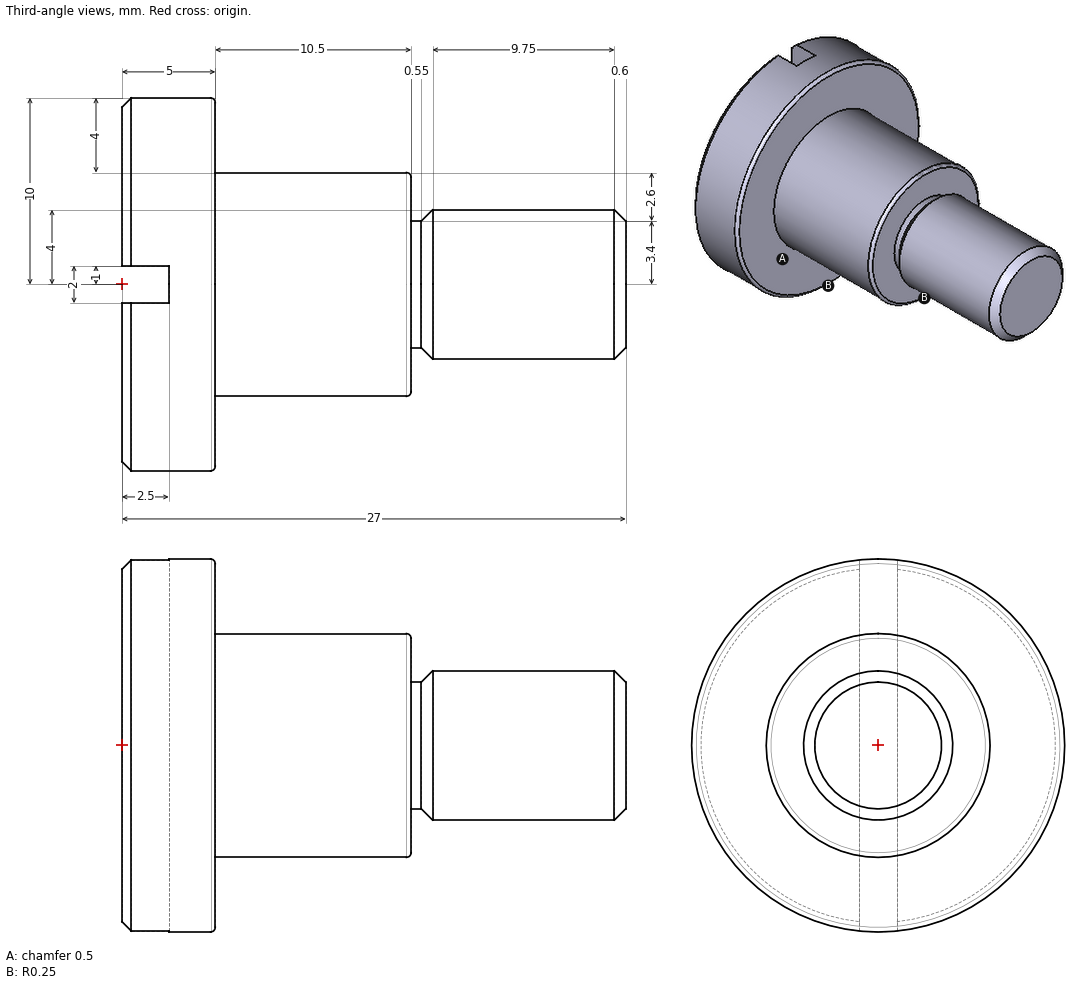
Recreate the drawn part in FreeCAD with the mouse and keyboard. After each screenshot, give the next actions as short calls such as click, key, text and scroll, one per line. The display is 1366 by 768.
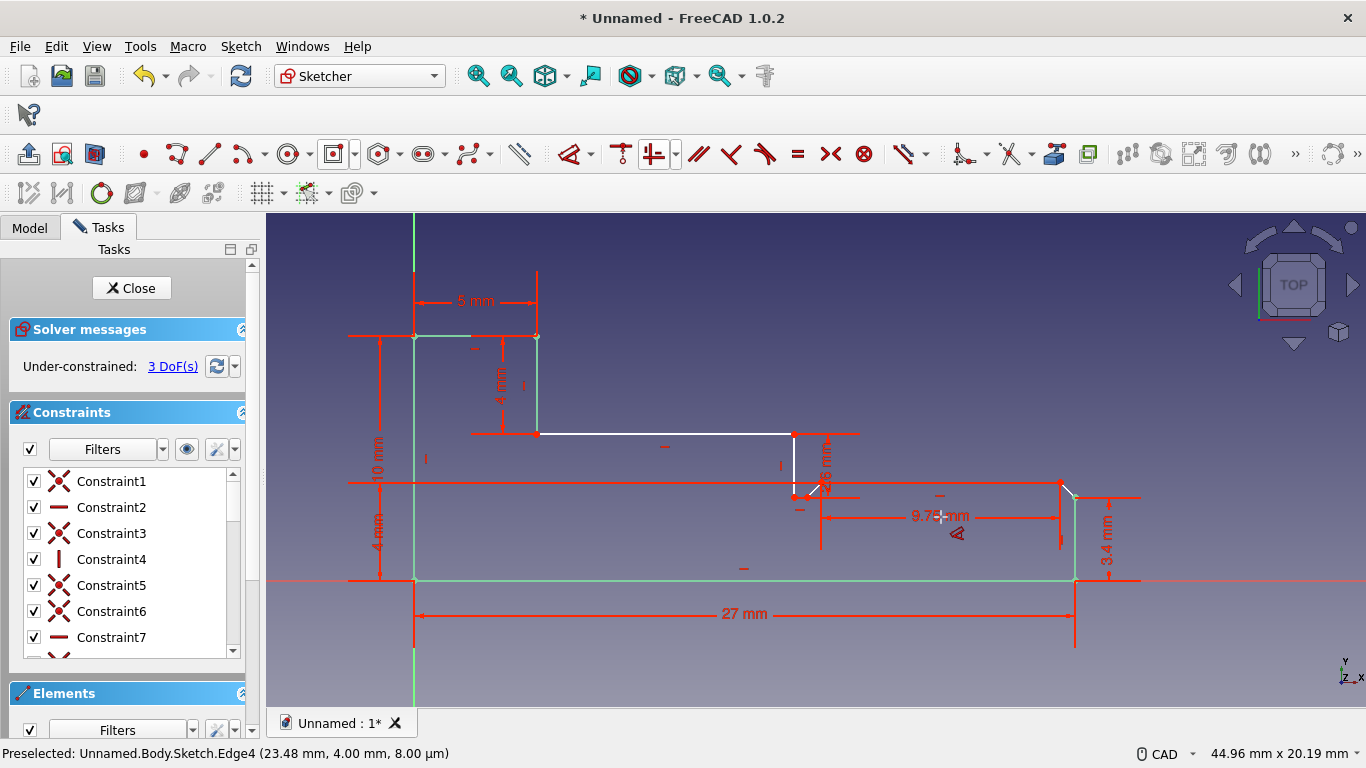
scroll(801, 498, up, 6)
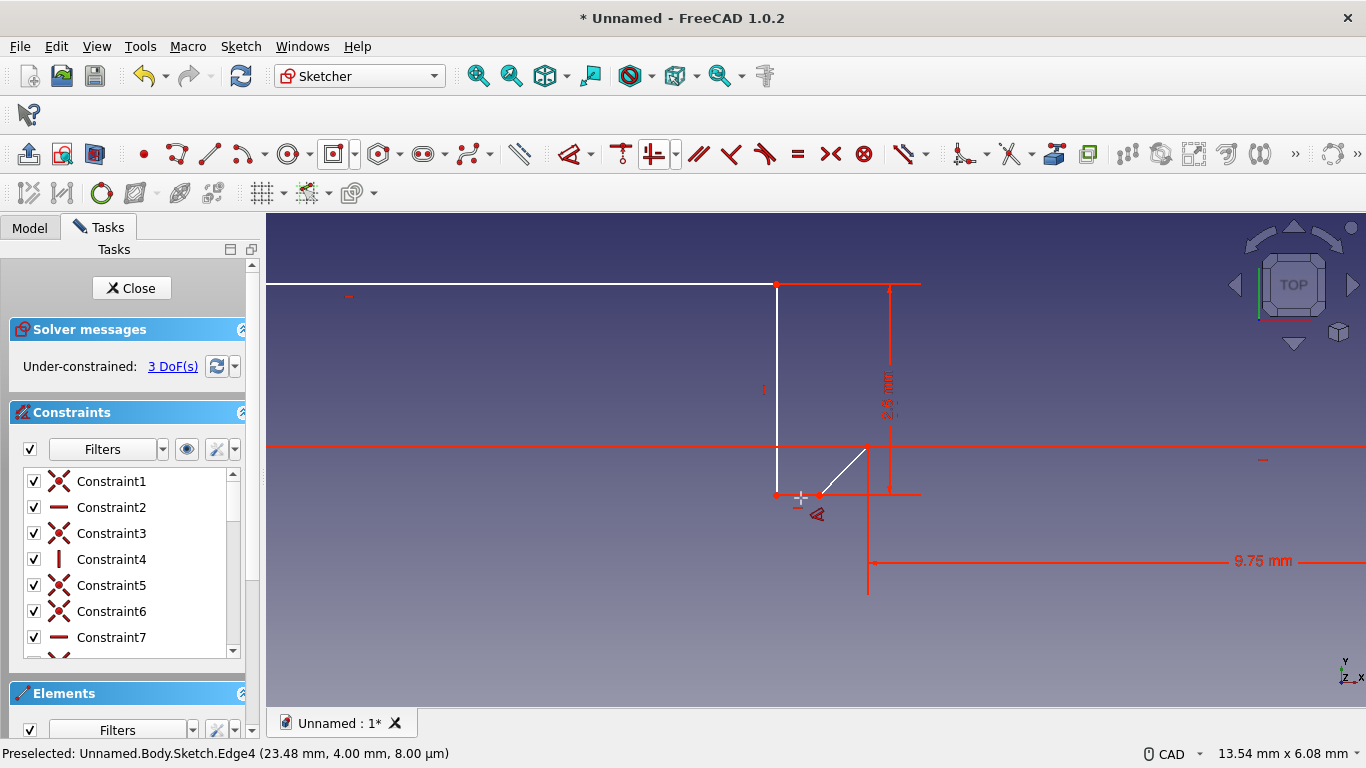
click(798, 495)
click(798, 529)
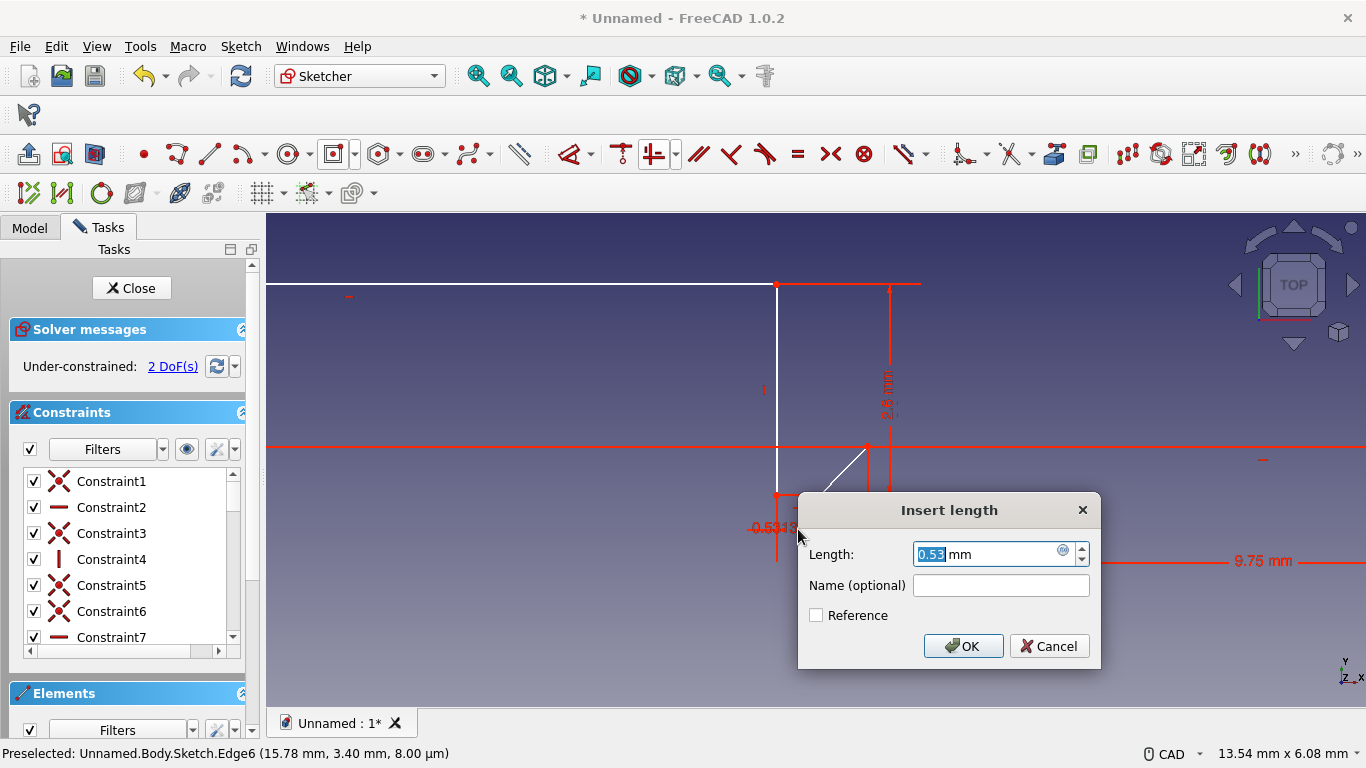
text(0.55)
key(Return)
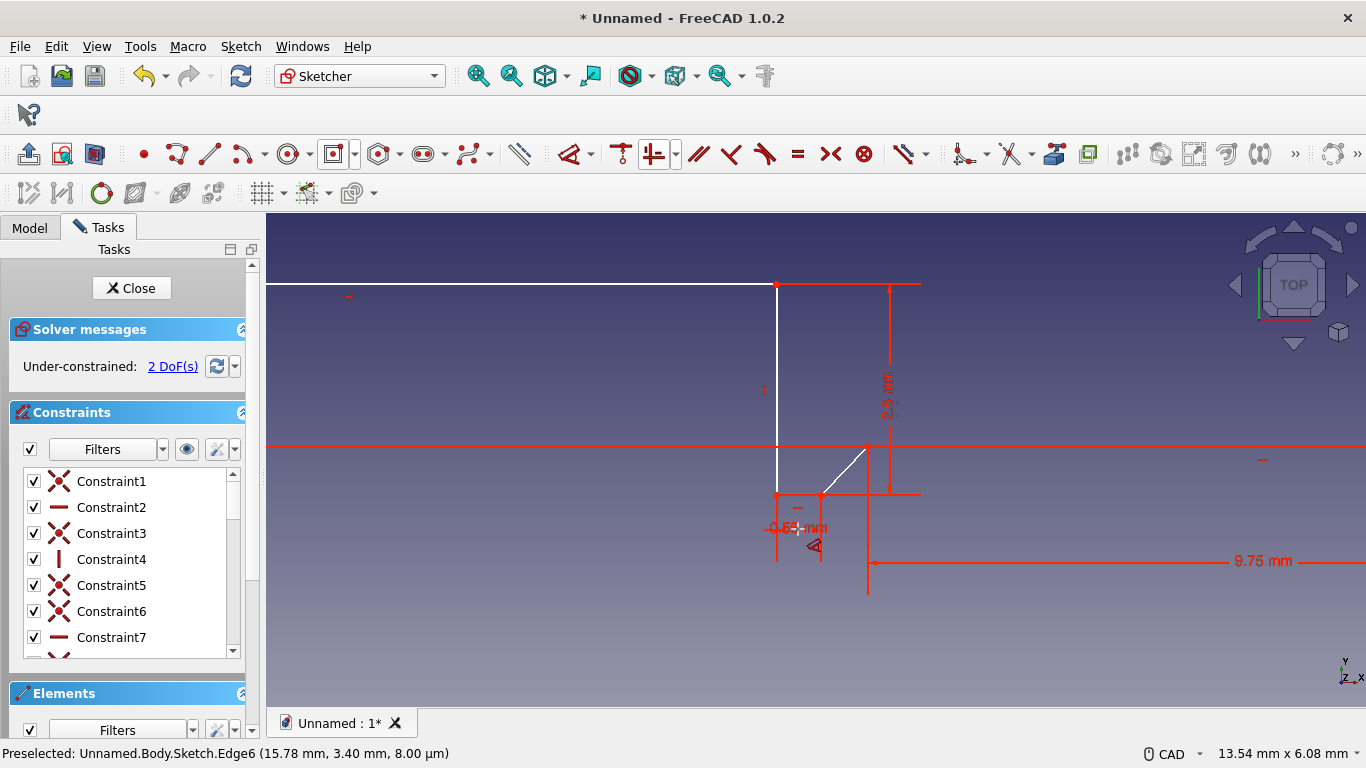
click(520, 284)
click(535, 250)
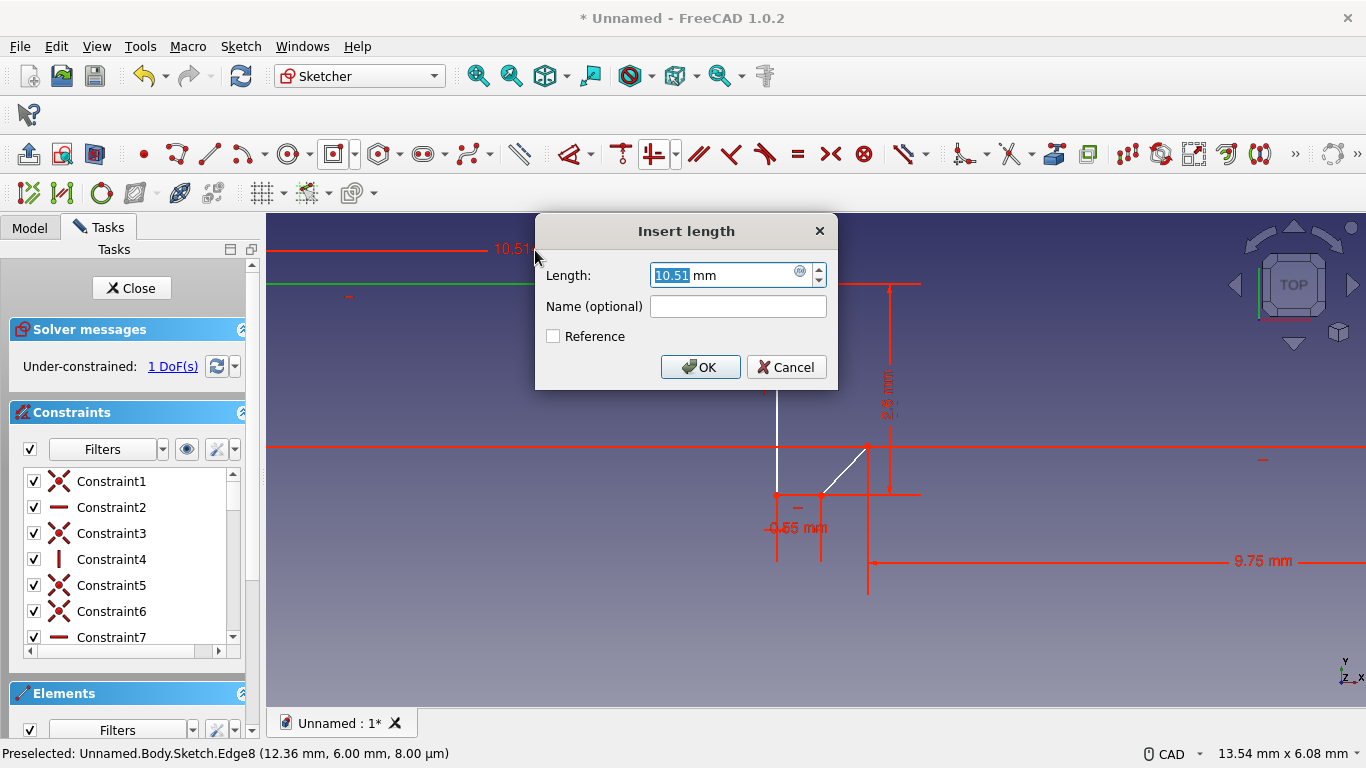
text(10.5)
key(Return)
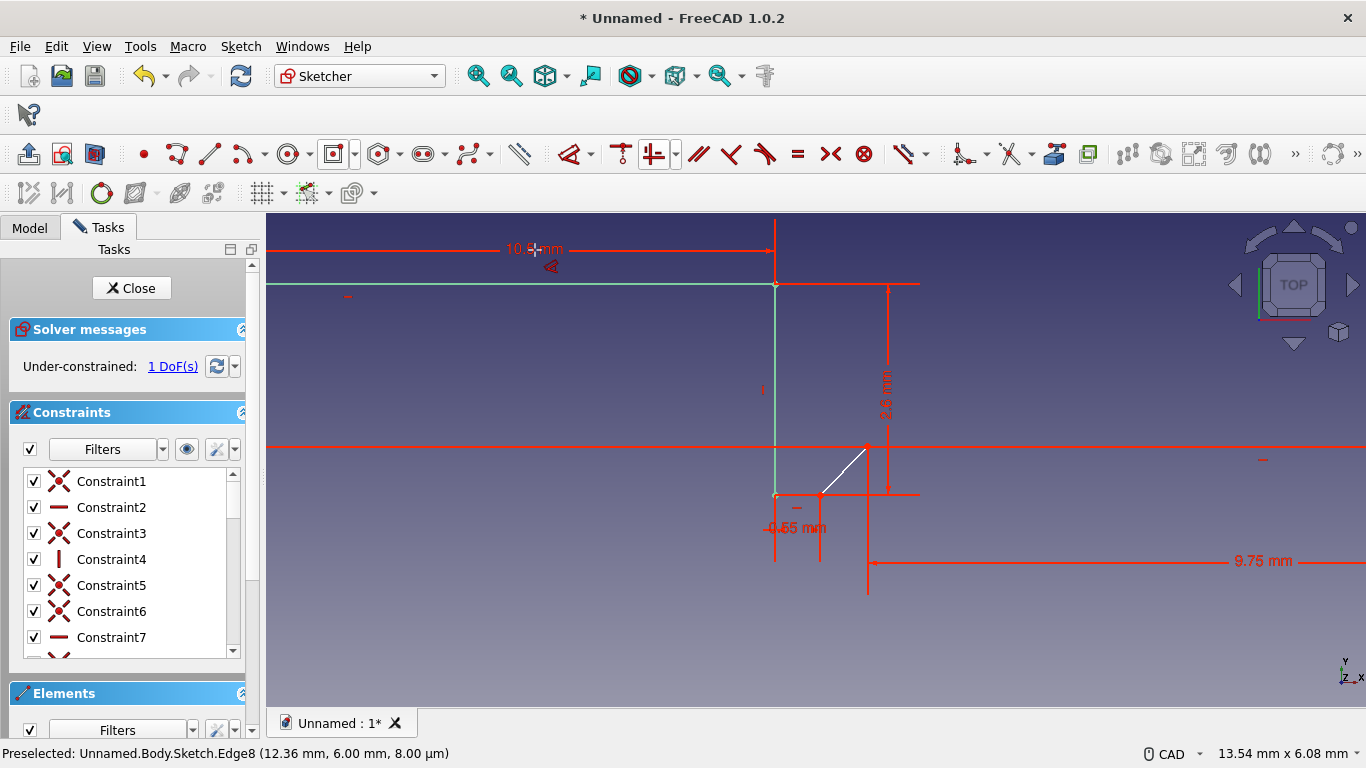
scroll(805, 501, down, 6)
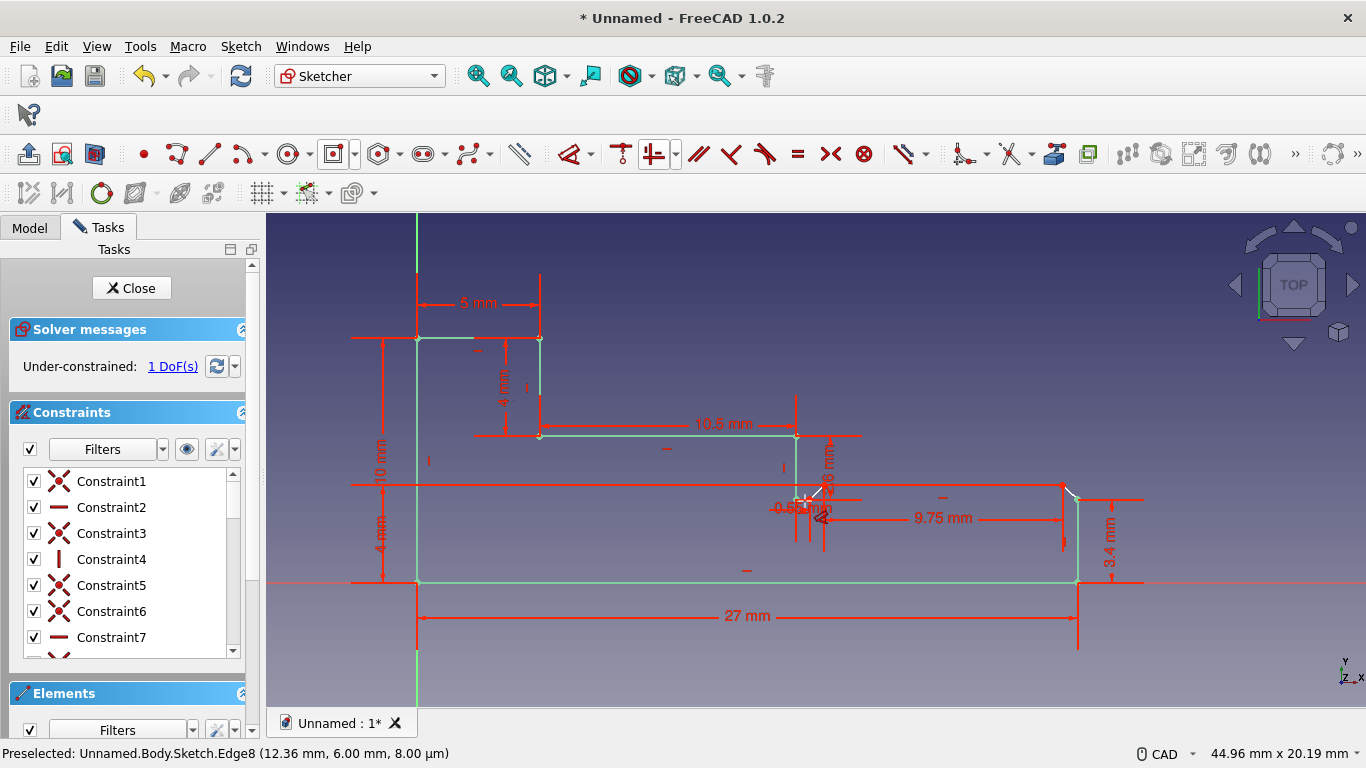
scroll(1073, 495, up, 5)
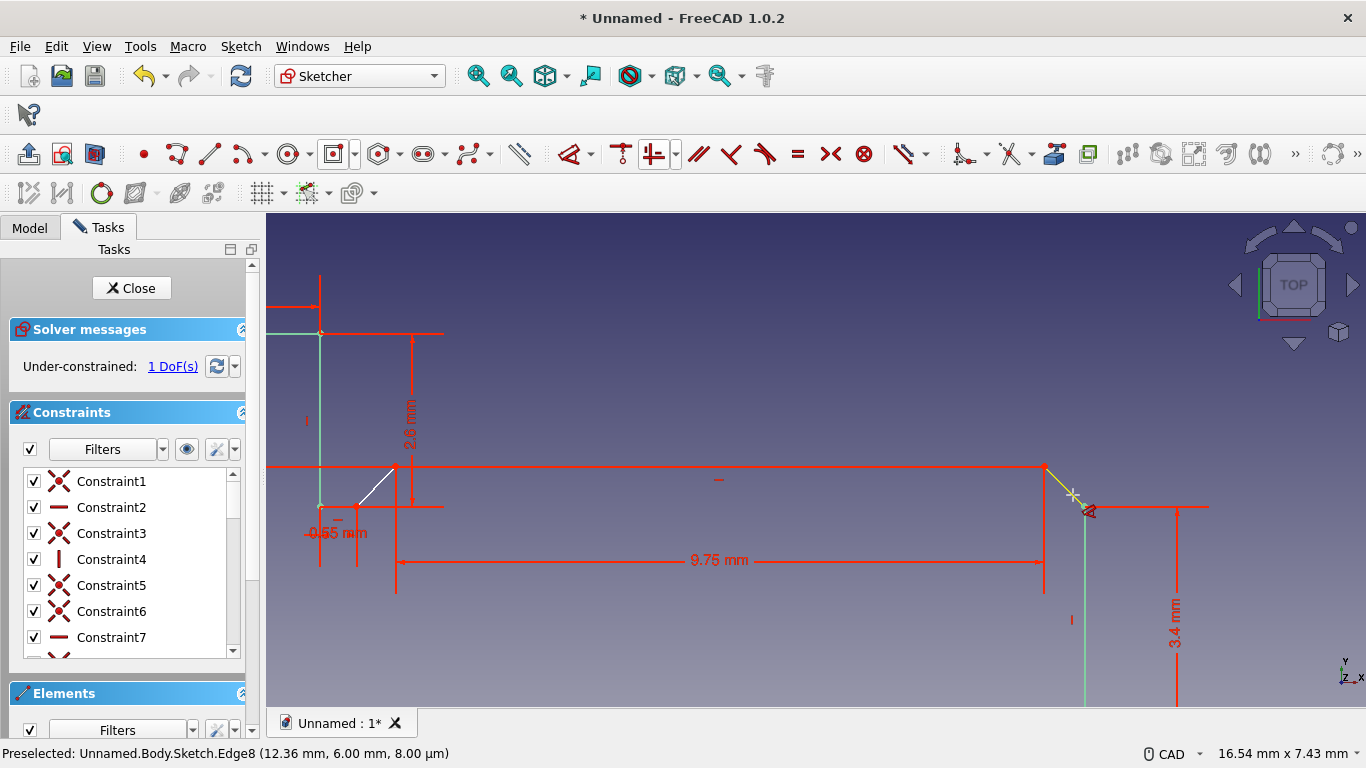
click(1073, 495)
click(1064, 541)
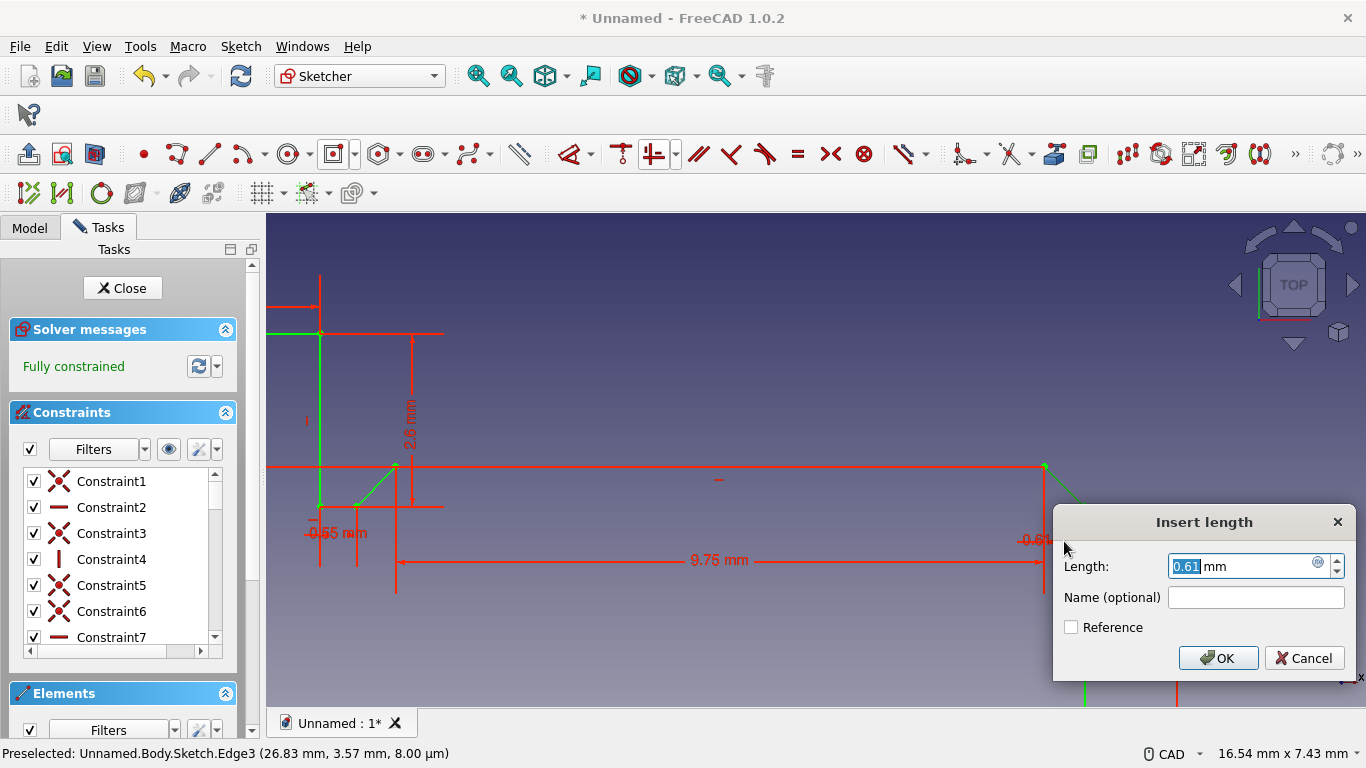
text(0.6)
key(Return)
key(Escape)